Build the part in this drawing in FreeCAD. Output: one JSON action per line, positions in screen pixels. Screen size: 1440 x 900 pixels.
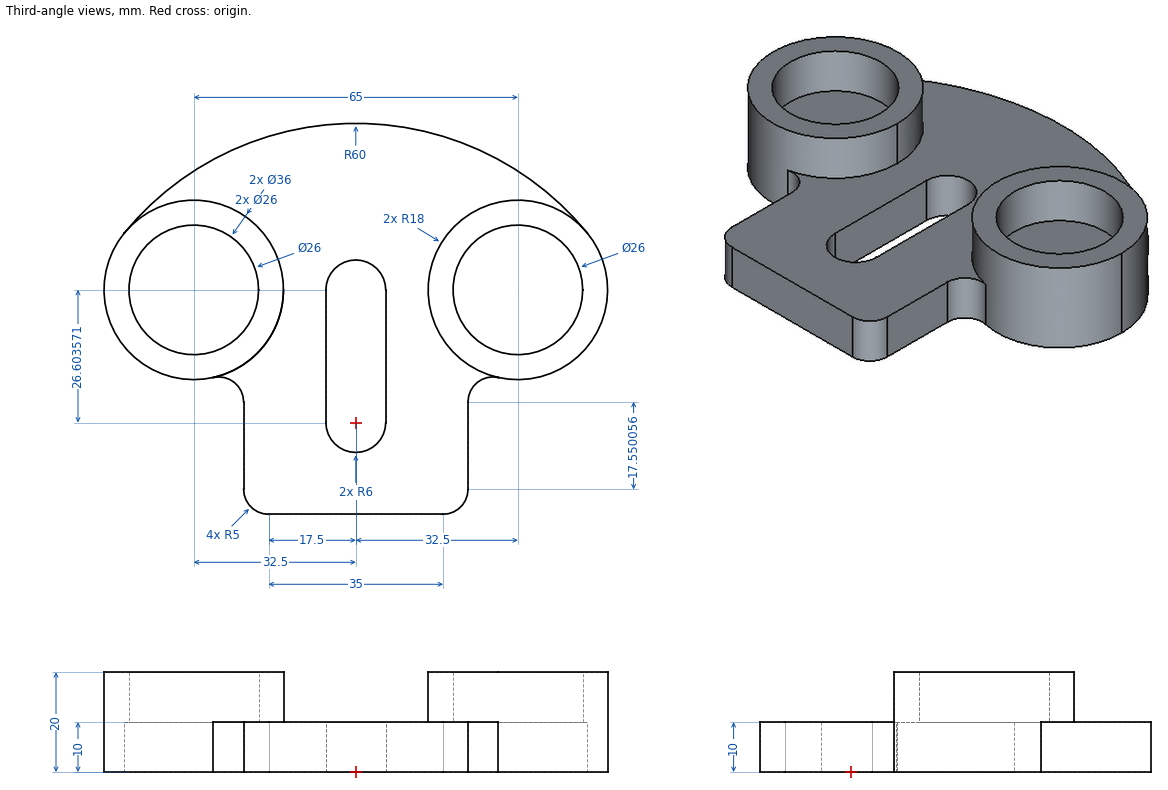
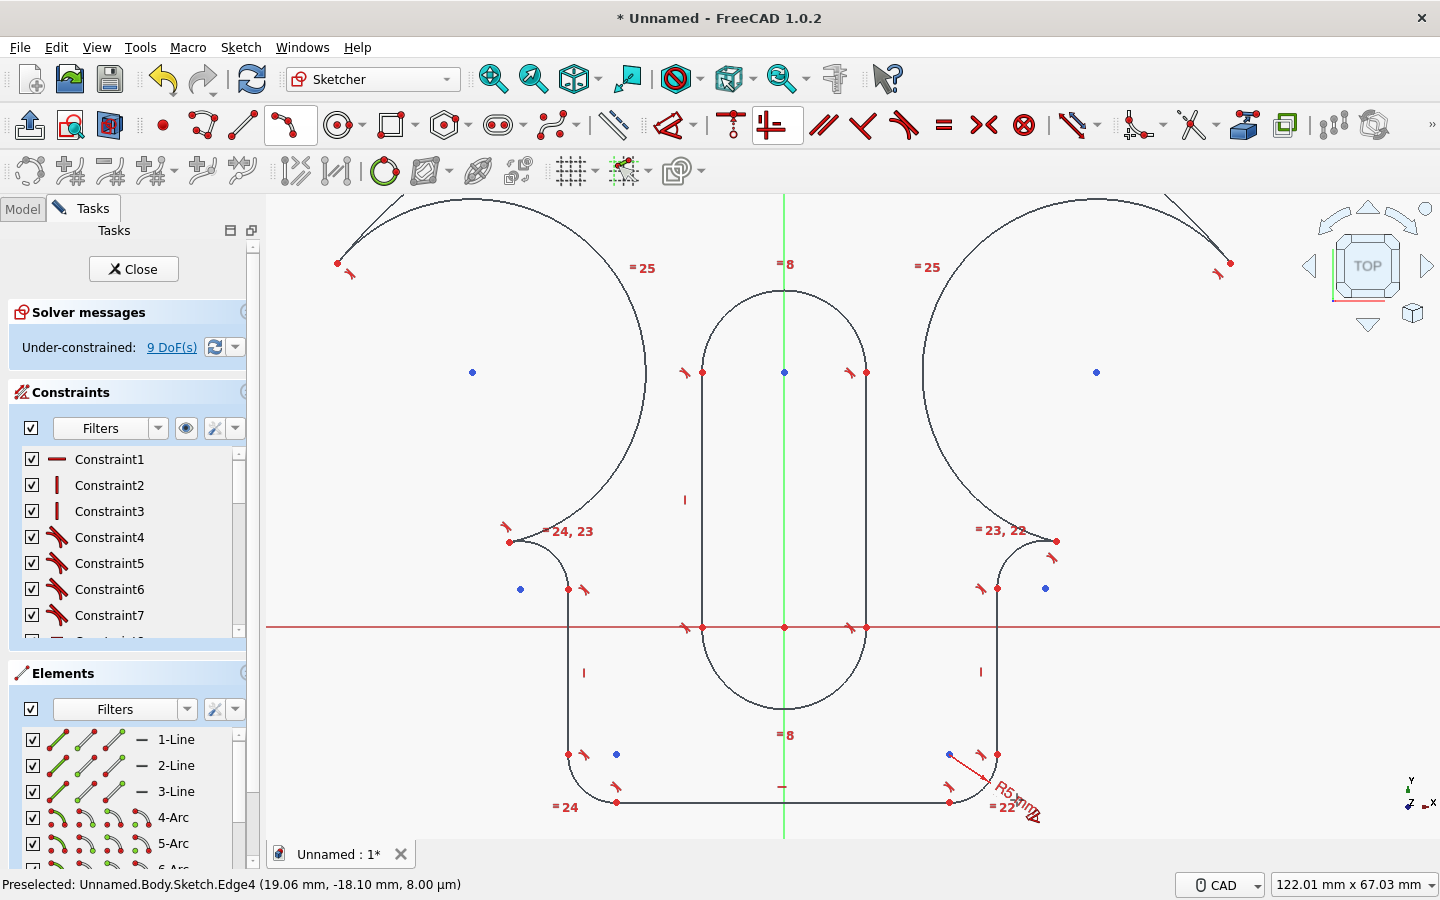
{"action": "left_click", "coordinate": [926, 407]}
{"action": "left_click", "coordinate": [895, 413]}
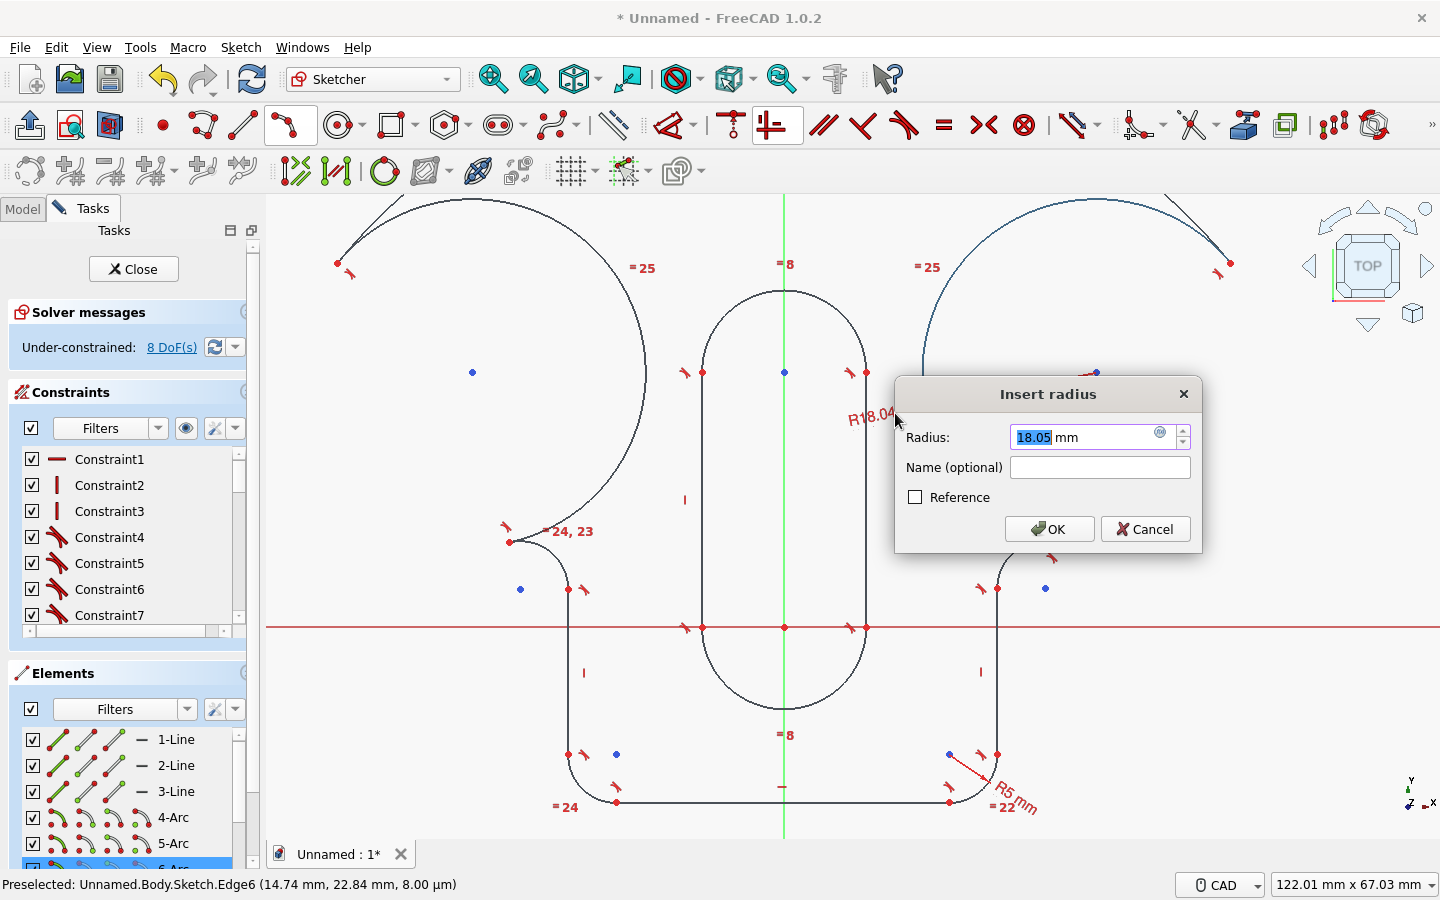
{"action": "type", "text": "18"}
{"action": "key", "text": "Return"}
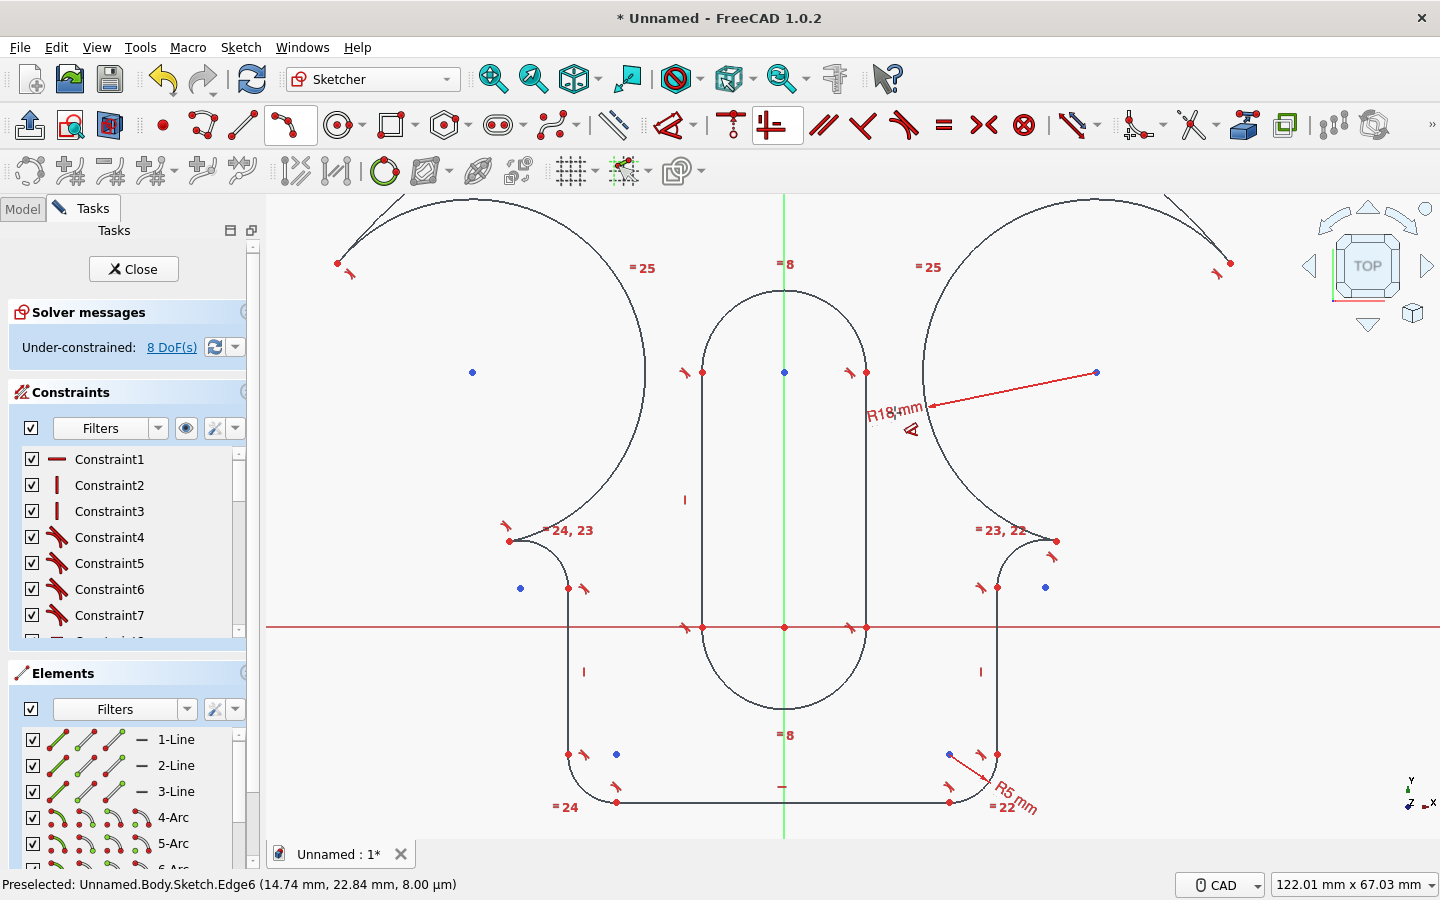
{"action": "scroll", "coordinate": [785, 625], "scroll_direction": "down", "scroll_amount": 3}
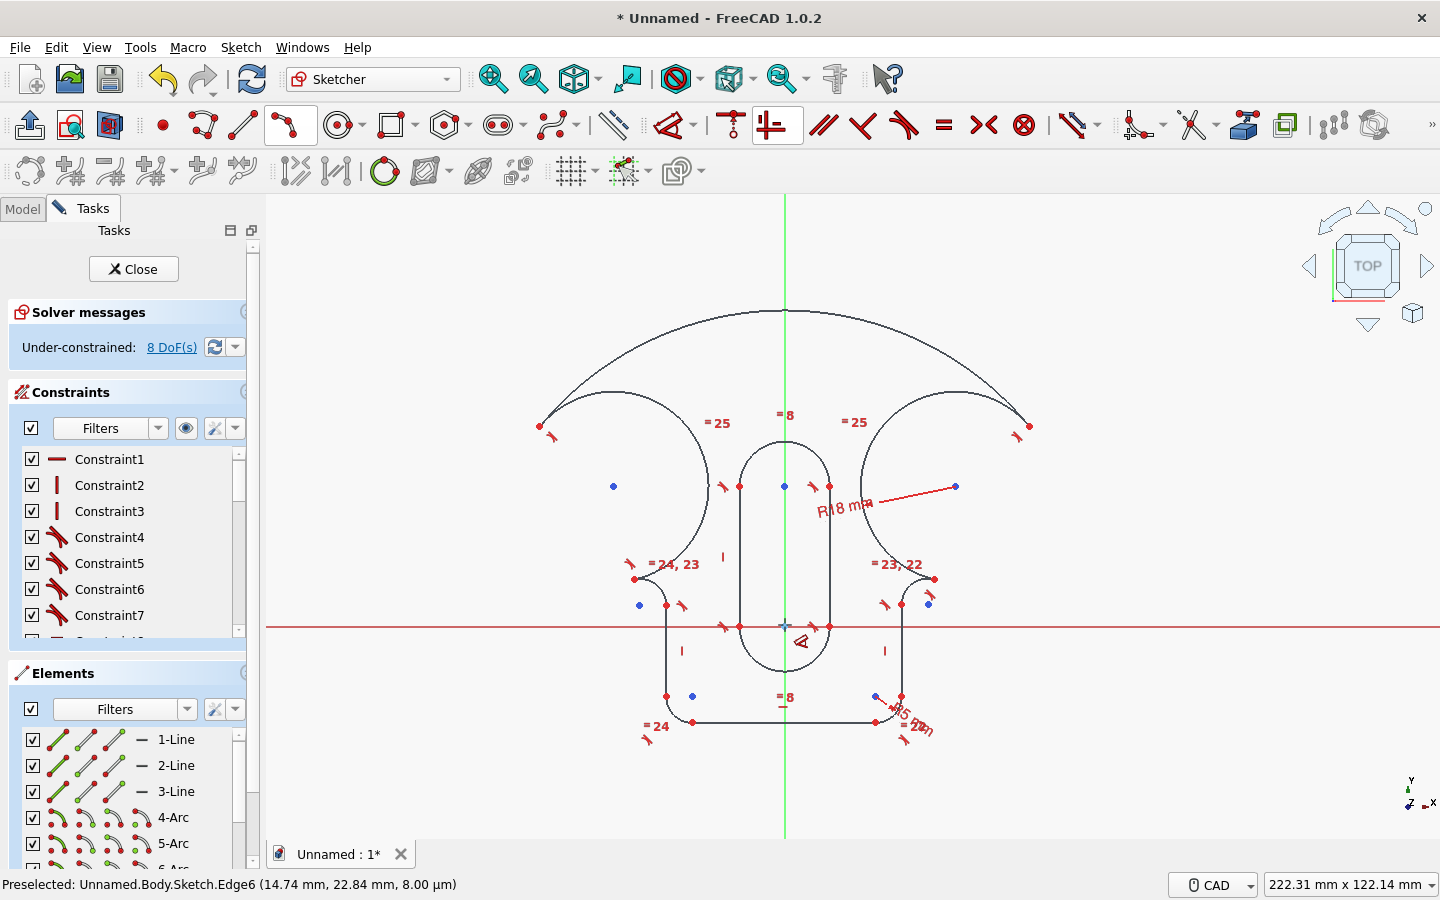
{"action": "left_click", "coordinate": [894, 330]}
{"action": "left_click", "coordinate": [905, 300]}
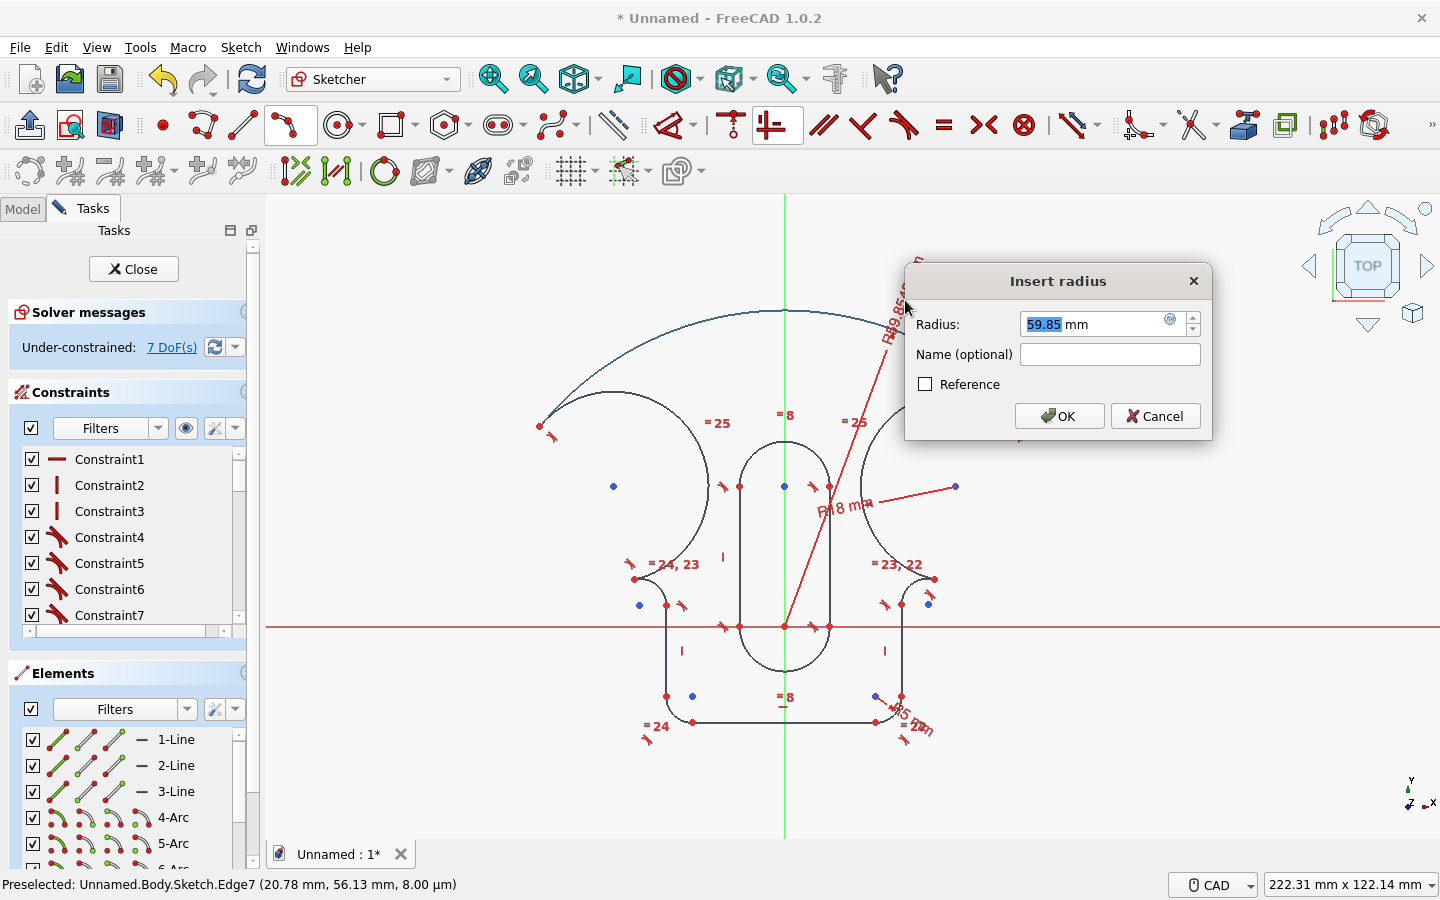
{"action": "type", "text": "60"}
{"action": "key", "text": "Return"}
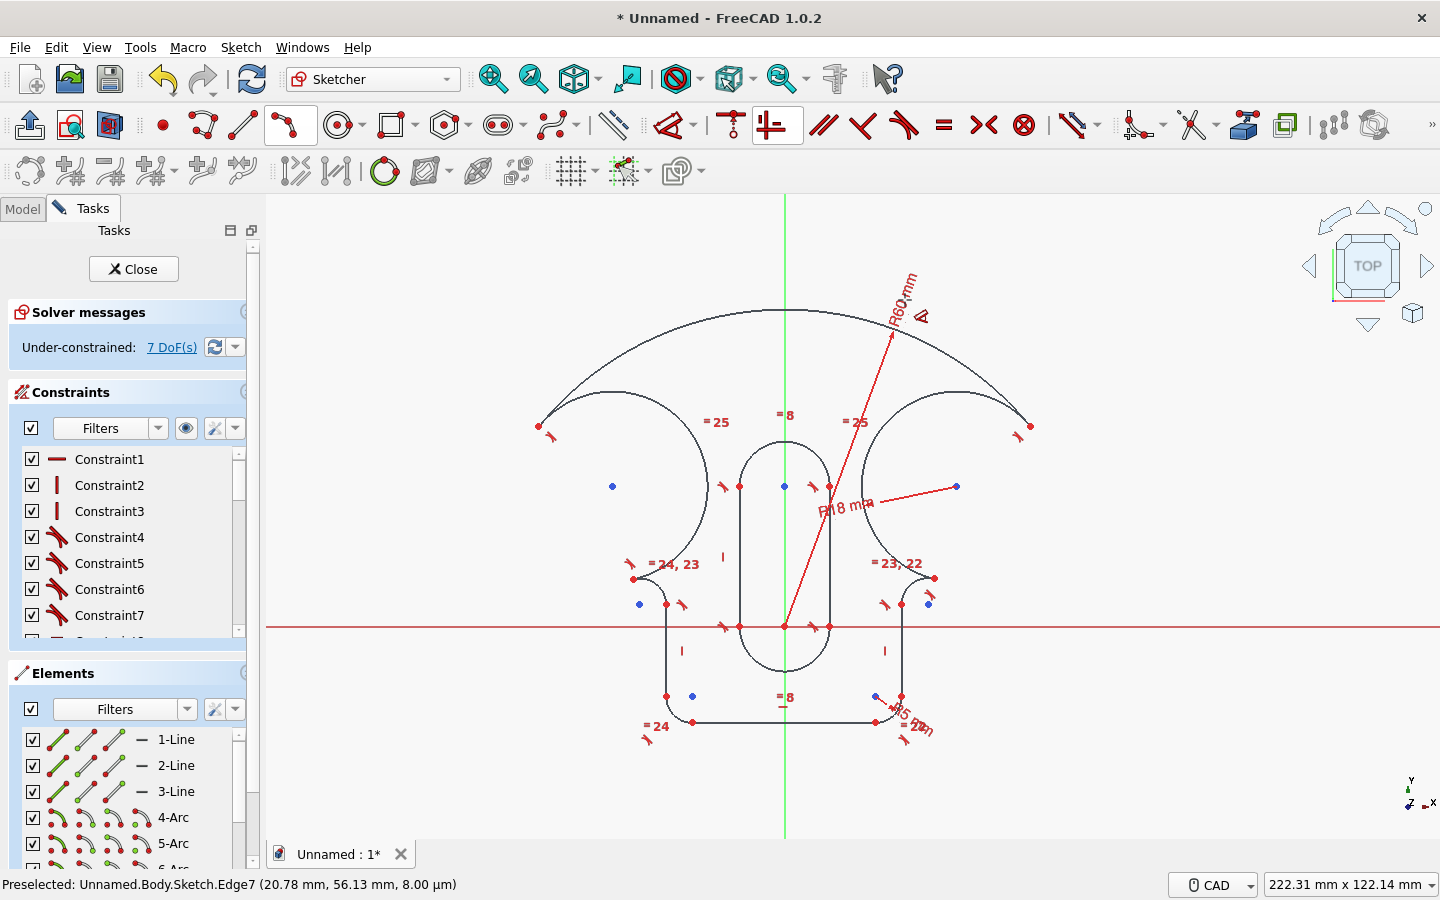
{"action": "scroll", "coordinate": [758, 663], "scroll_direction": "up", "scroll_amount": 2}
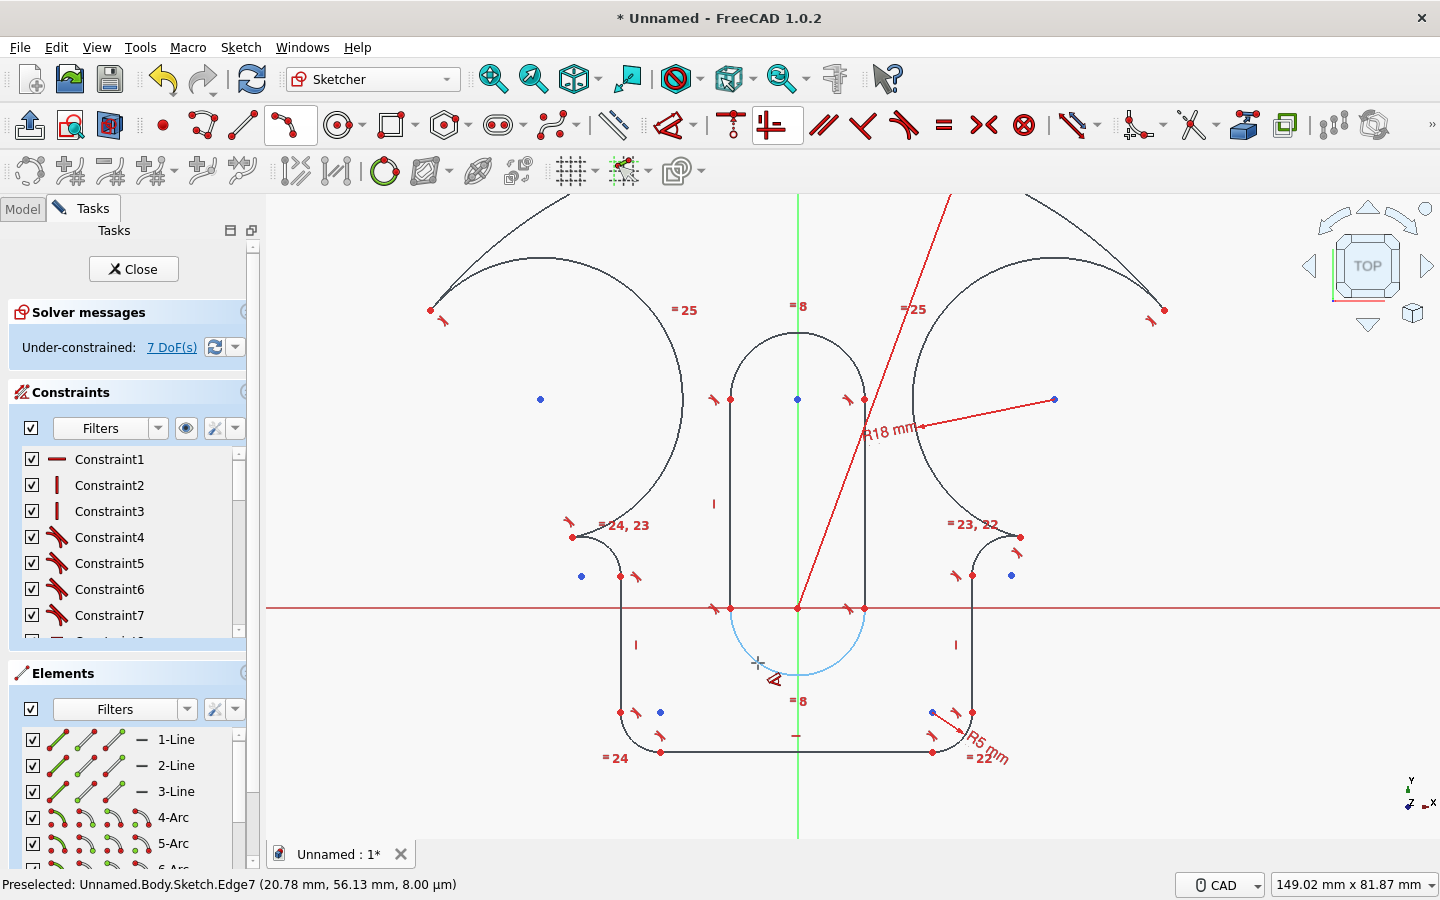
{"action": "left_click", "coordinate": [758, 663]}
{"action": "left_click", "coordinate": [739, 689]}